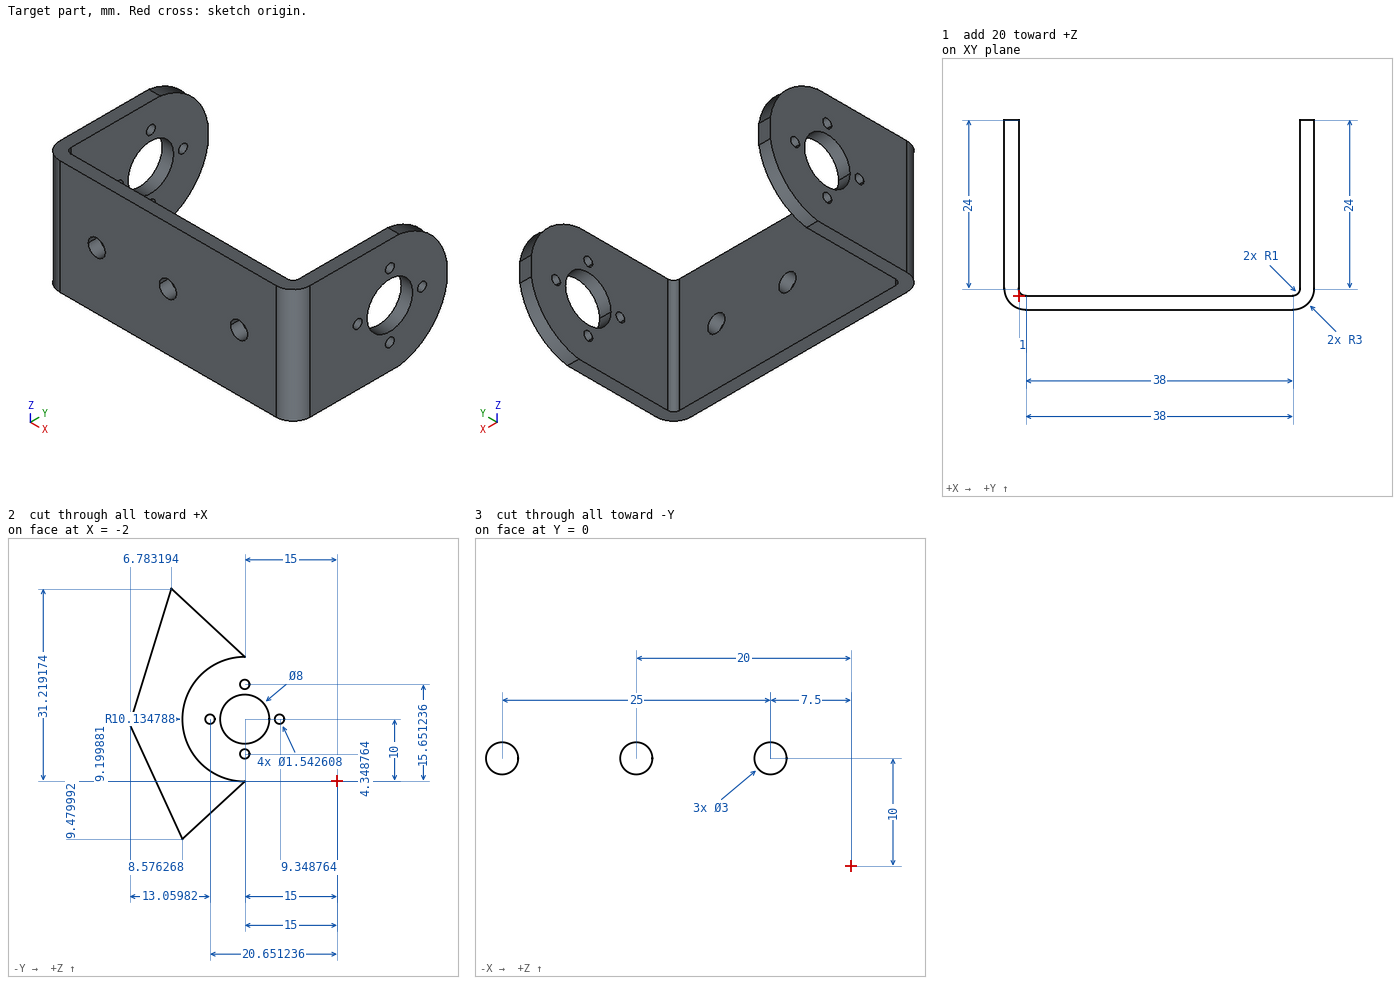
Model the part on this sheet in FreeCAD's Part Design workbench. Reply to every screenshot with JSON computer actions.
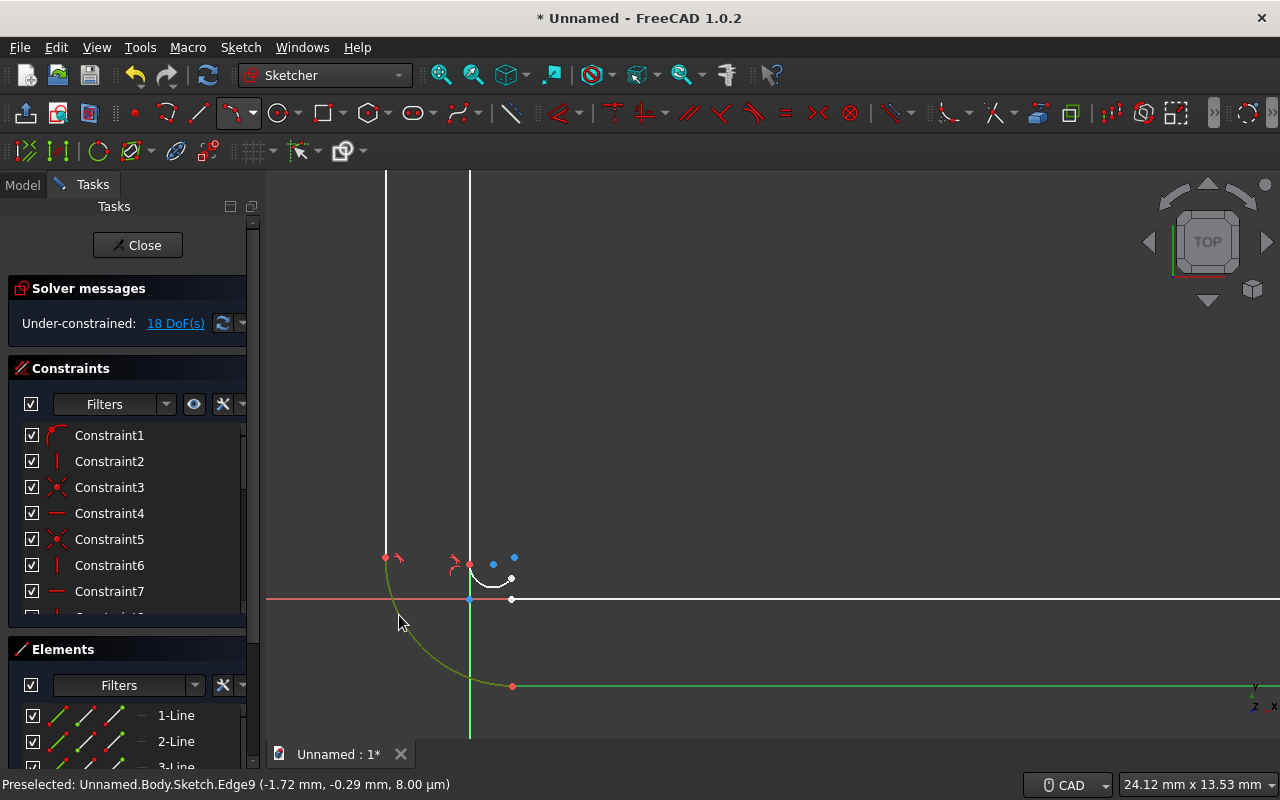
{"action": "key", "text": "t"}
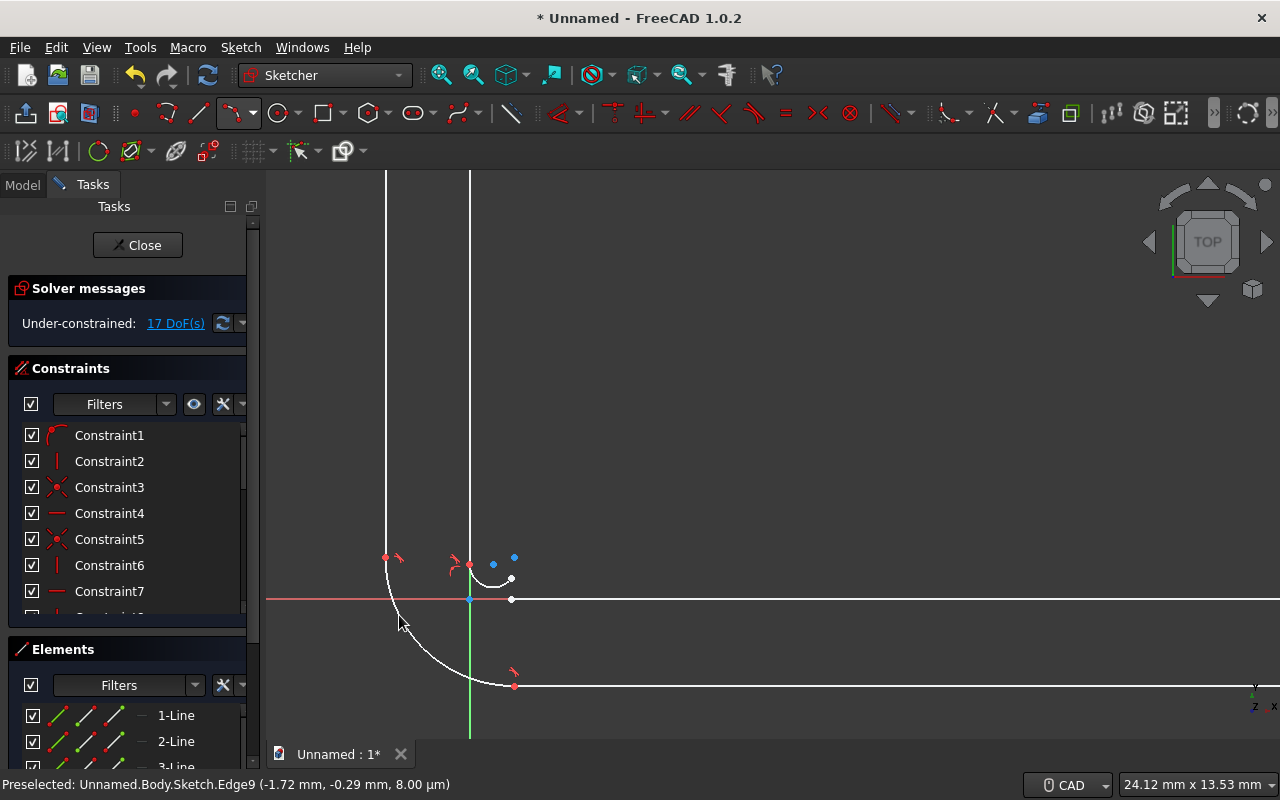
{"action": "left_click", "coordinate": [993, 686]}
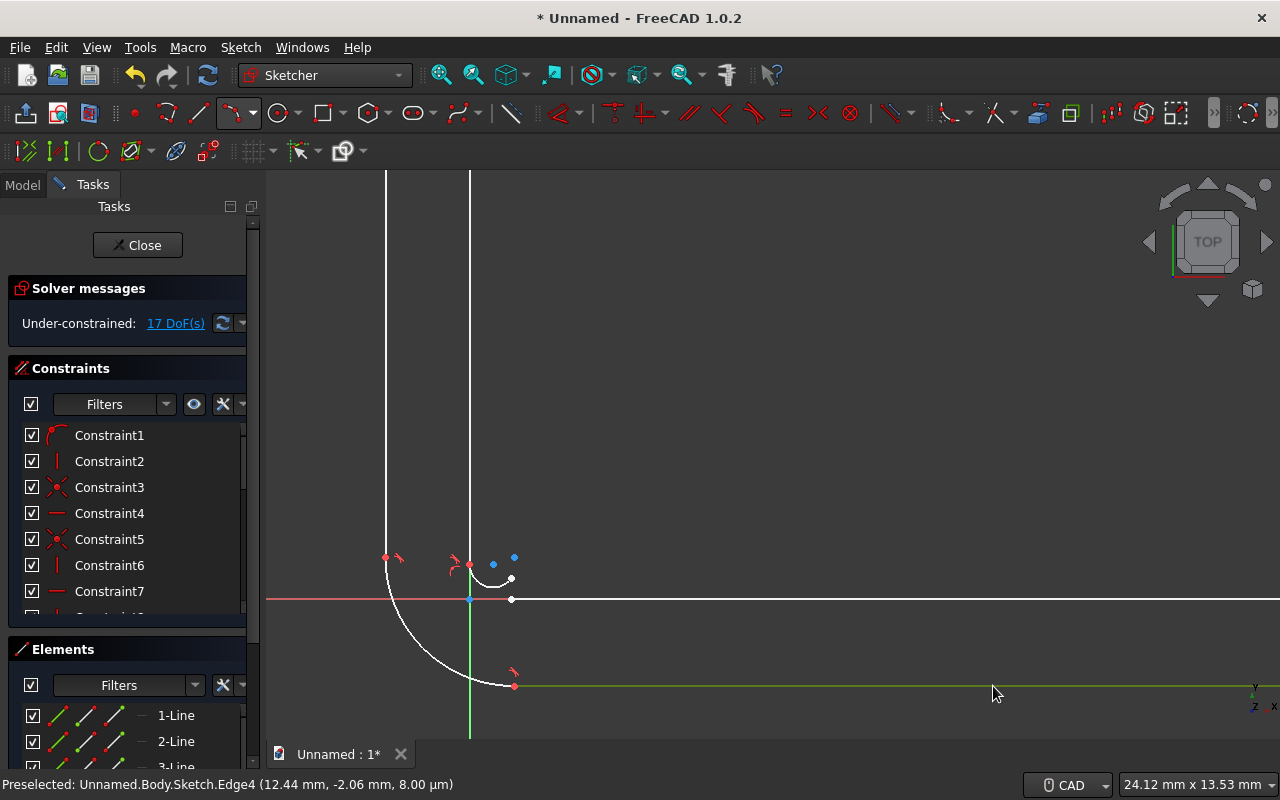
{"action": "scroll", "coordinate": [443, 600], "scroll_direction": "down", "scroll_amount": 6}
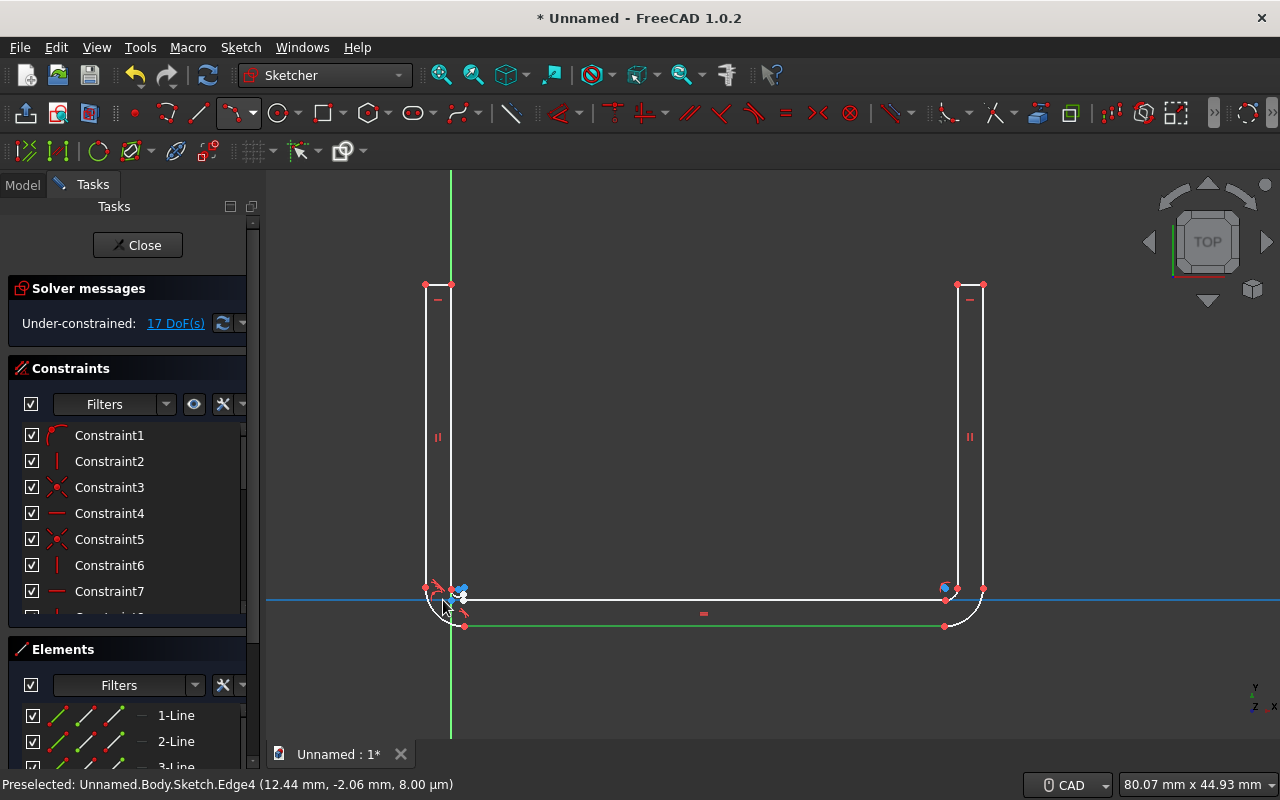
{"action": "left_click", "coordinate": [962, 622]}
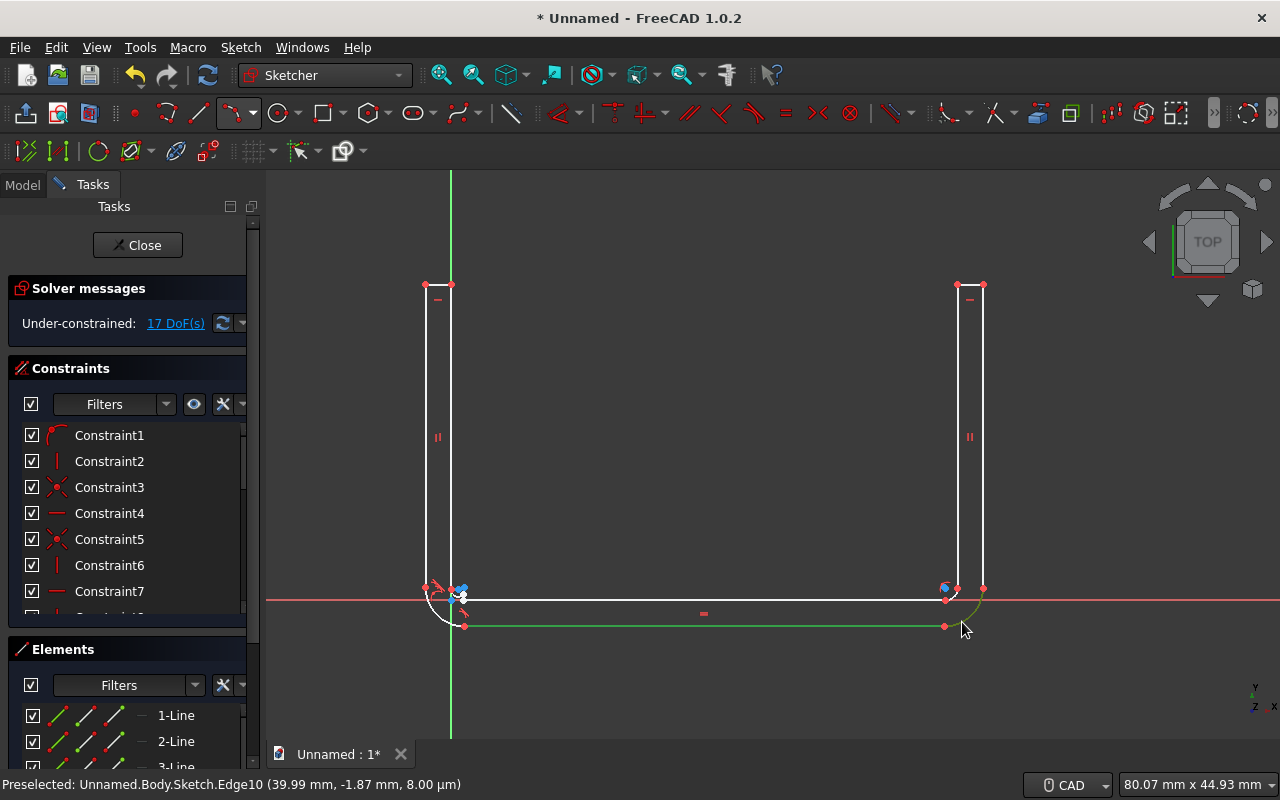
{"action": "key", "text": "t"}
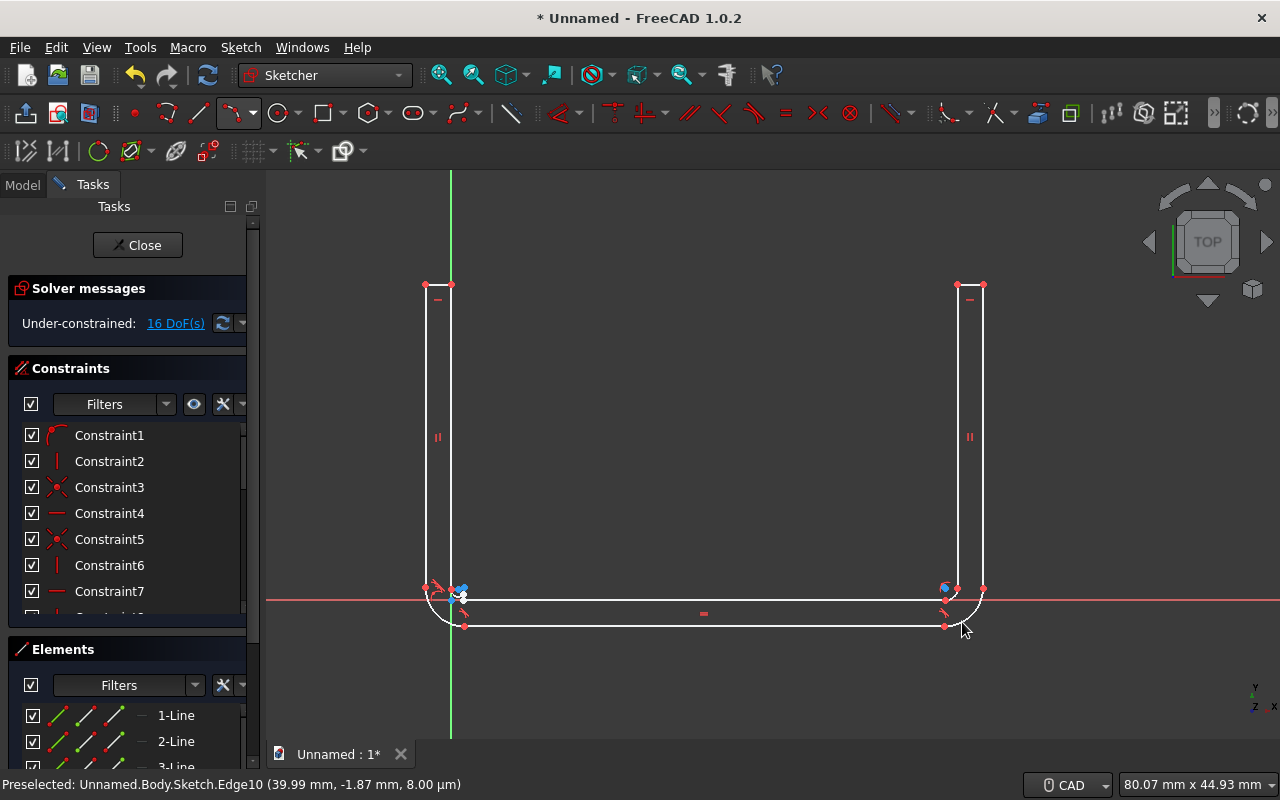
{"action": "left_click", "coordinate": [983, 497]}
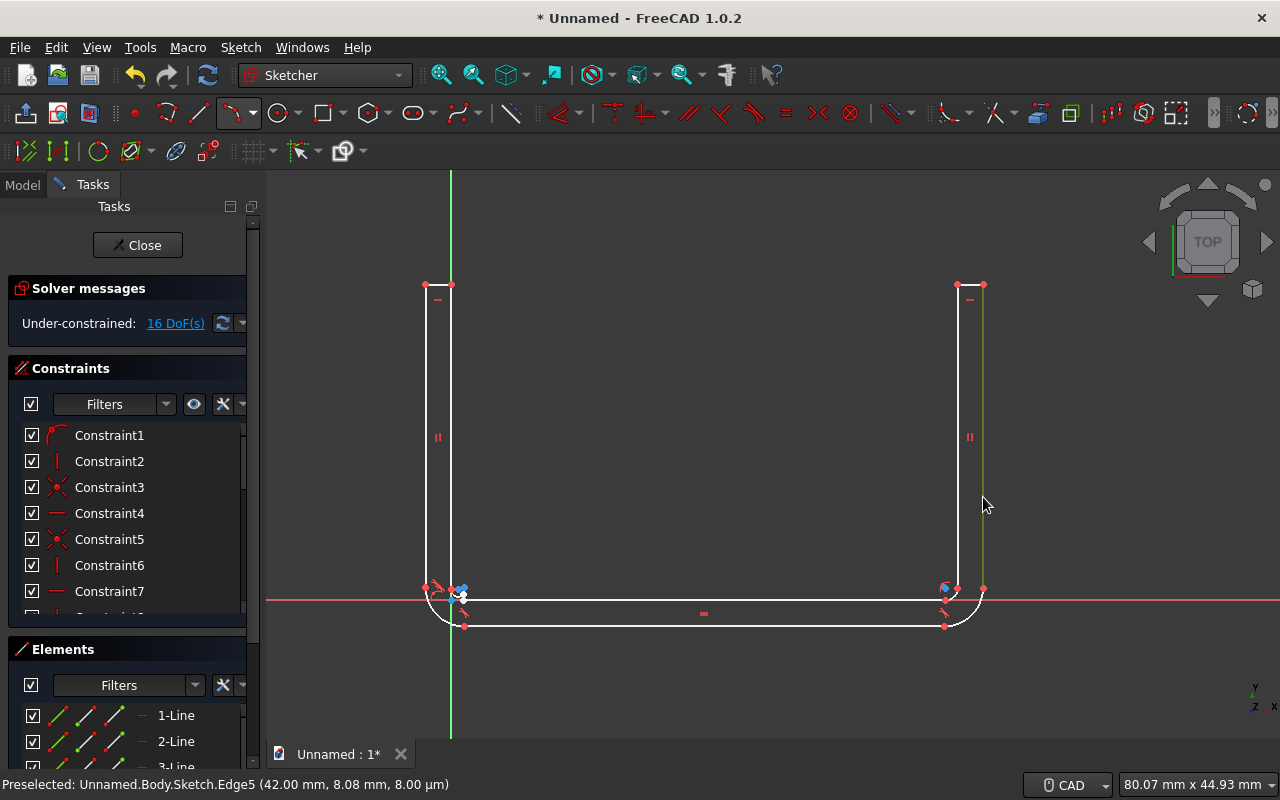
{"action": "left_click", "coordinate": [962, 622]}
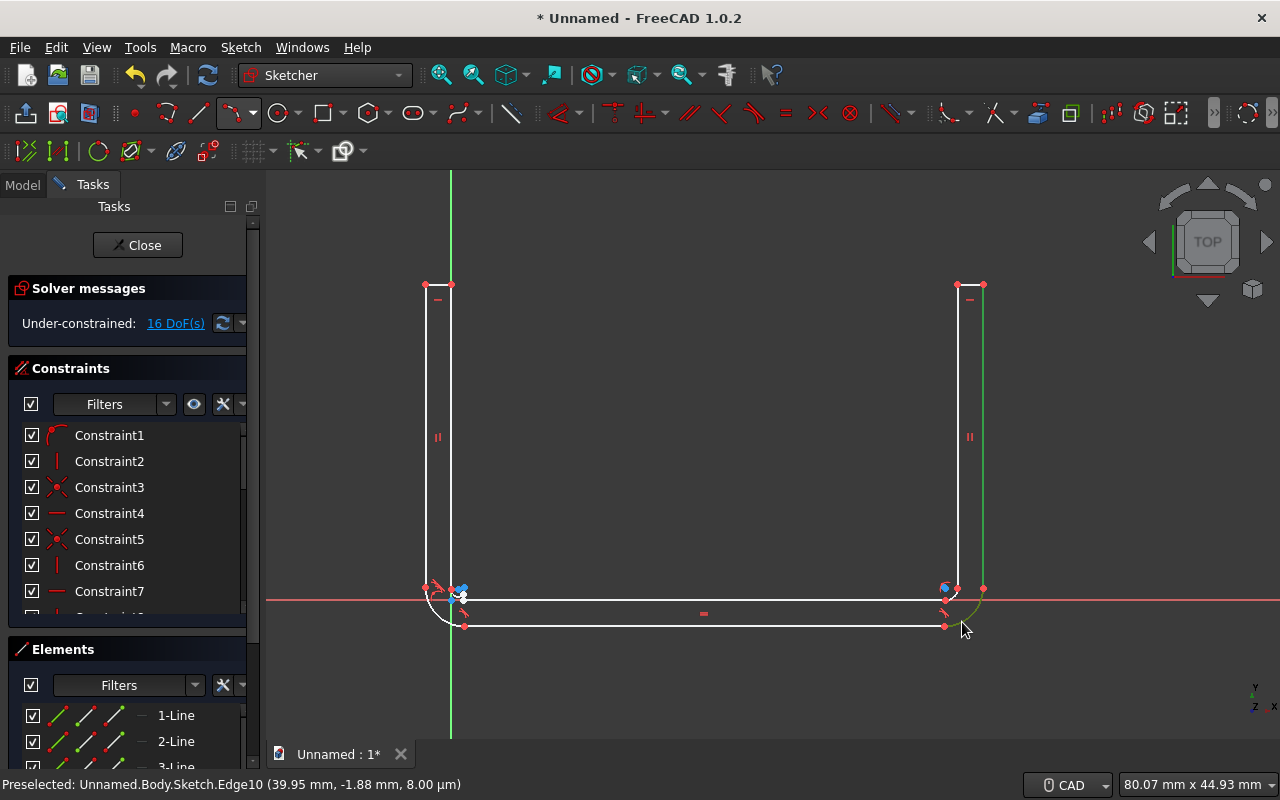
{"action": "left_click", "coordinate": [754, 114]}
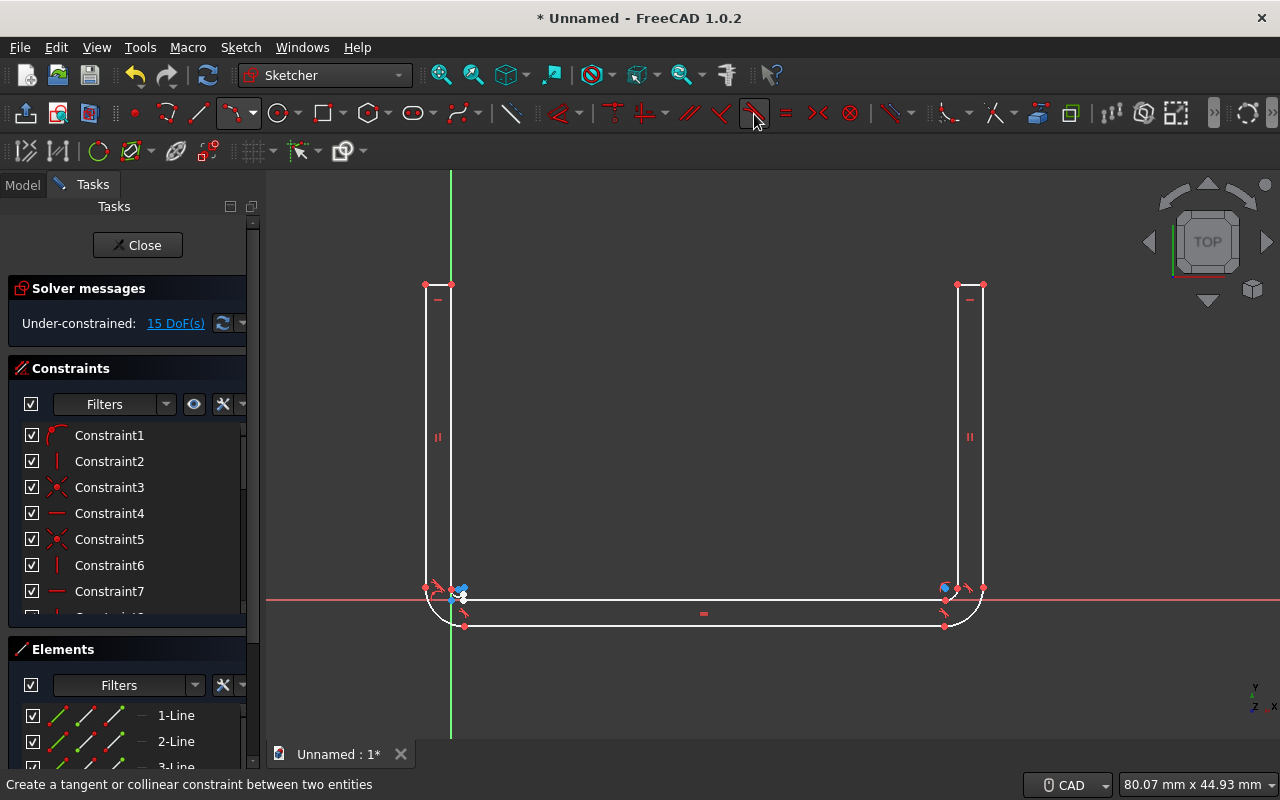
{"action": "left_click", "coordinate": [958, 376]}